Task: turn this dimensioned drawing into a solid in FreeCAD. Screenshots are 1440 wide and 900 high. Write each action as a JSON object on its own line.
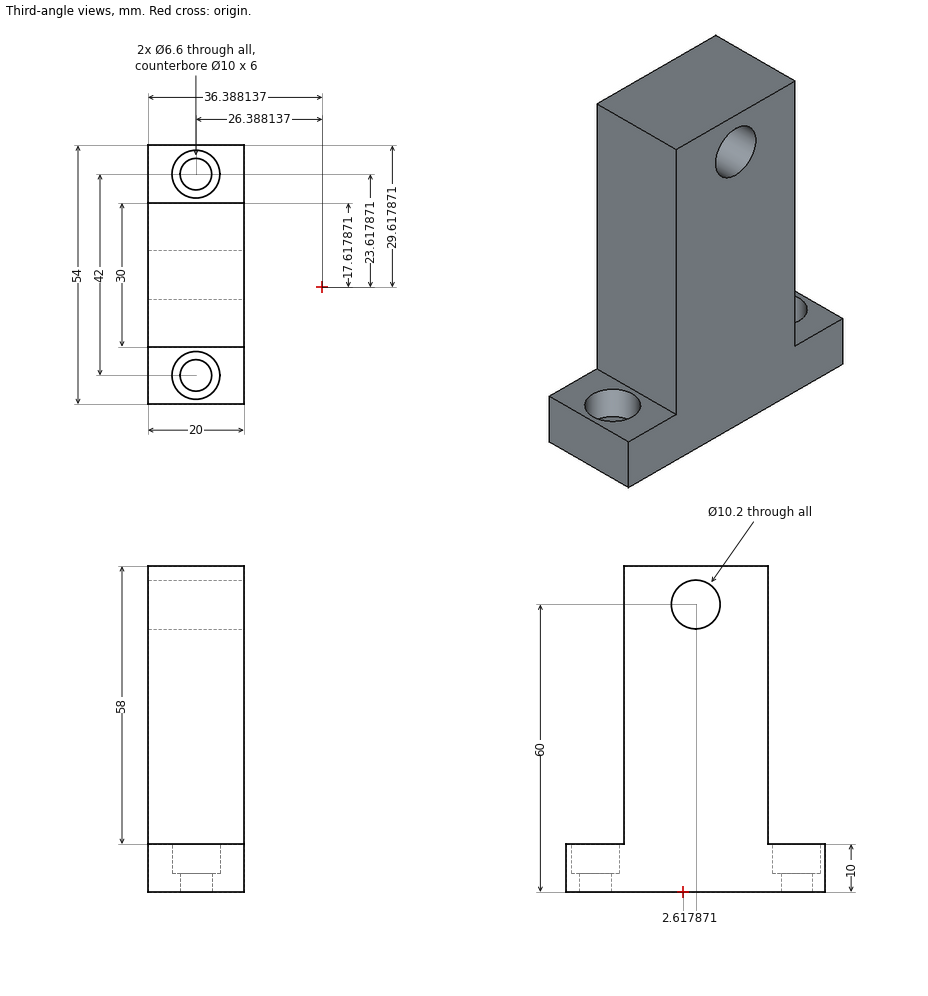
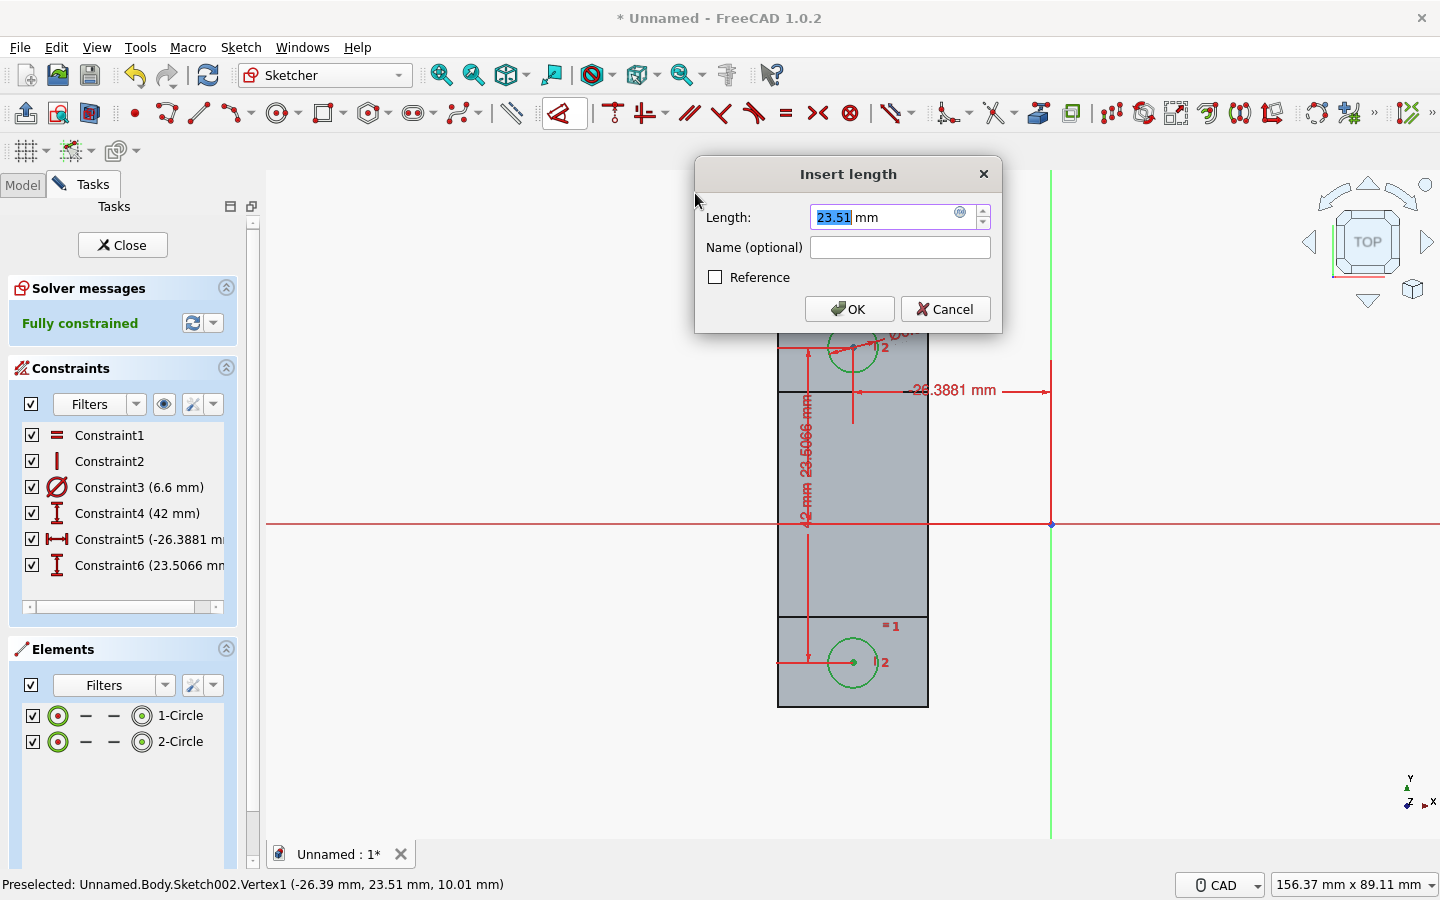
{"action": "type", "text": "23.617871"}
{"action": "key", "text": "Return"}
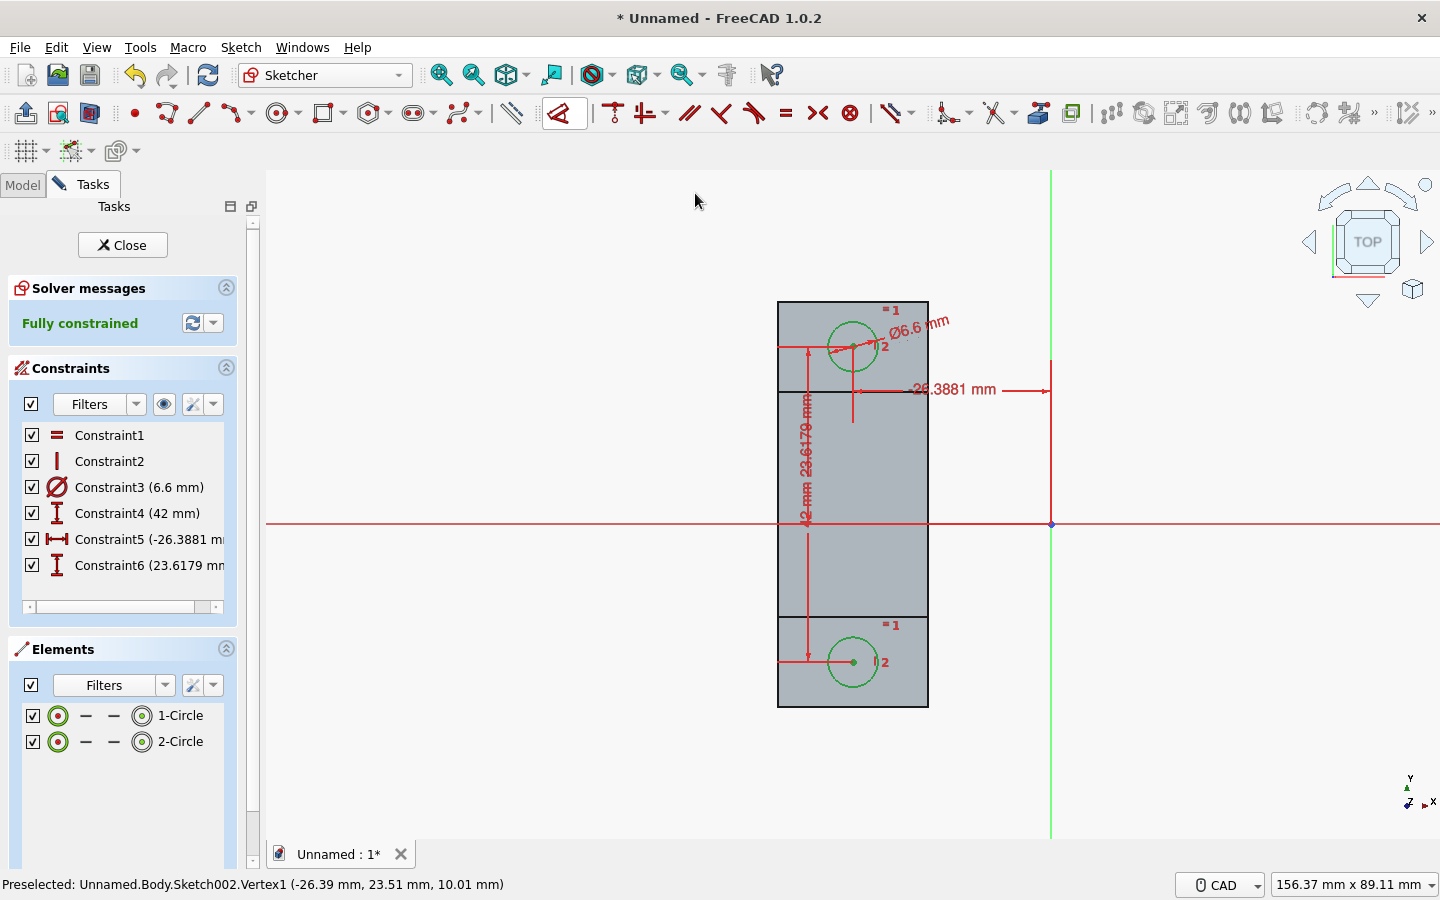
{"action": "left_click", "coordinate": [123, 245]}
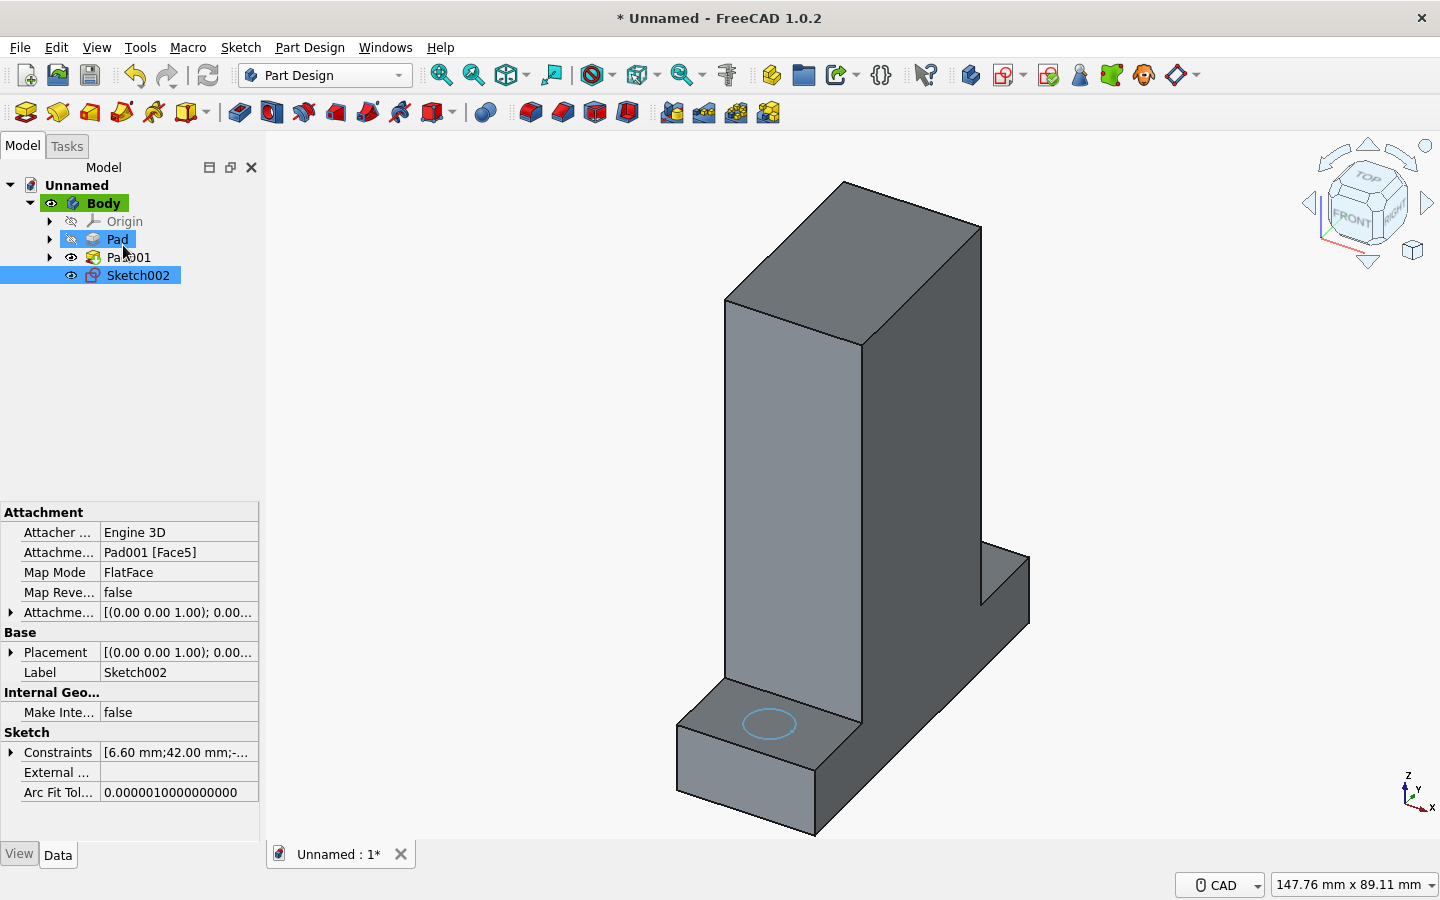
{"action": "left_click", "coordinate": [272, 112]}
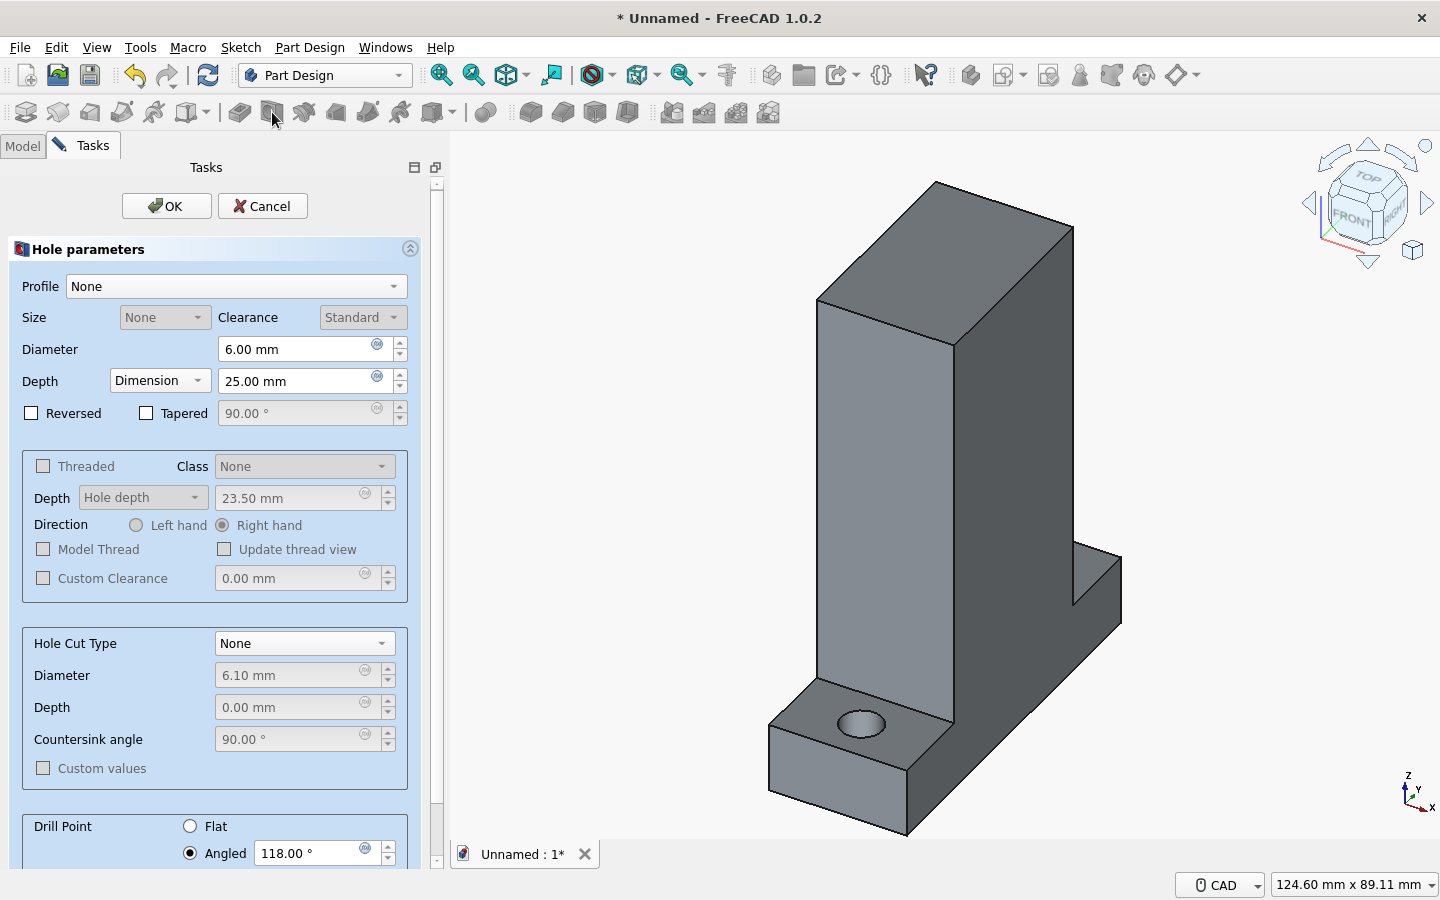
{"action": "triple_click", "coordinate": [305, 349]}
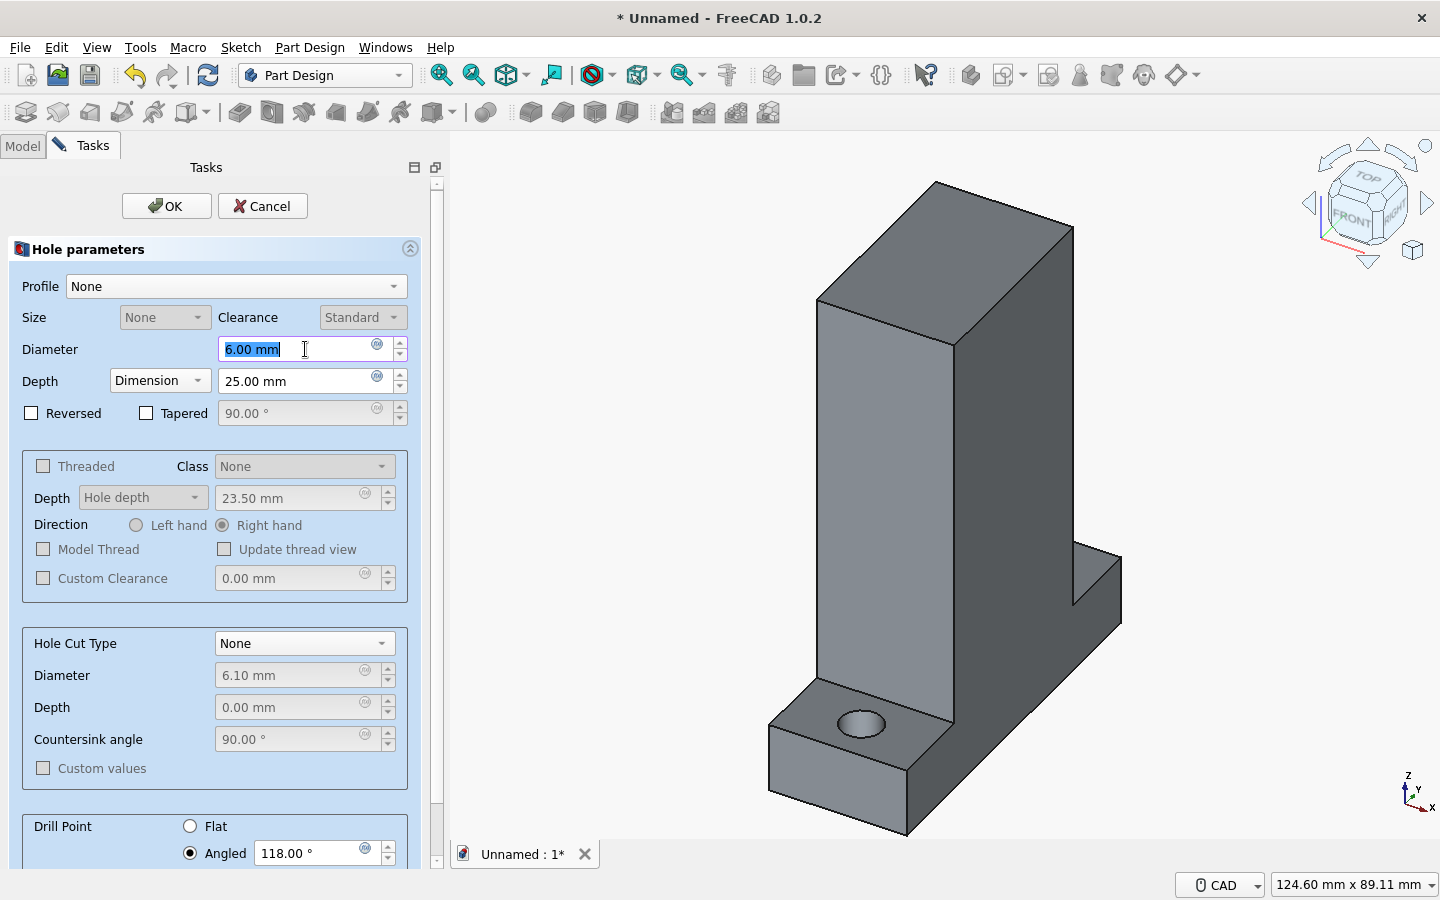
{"action": "type", "text": "6.6"}
{"action": "key", "text": "Tab"}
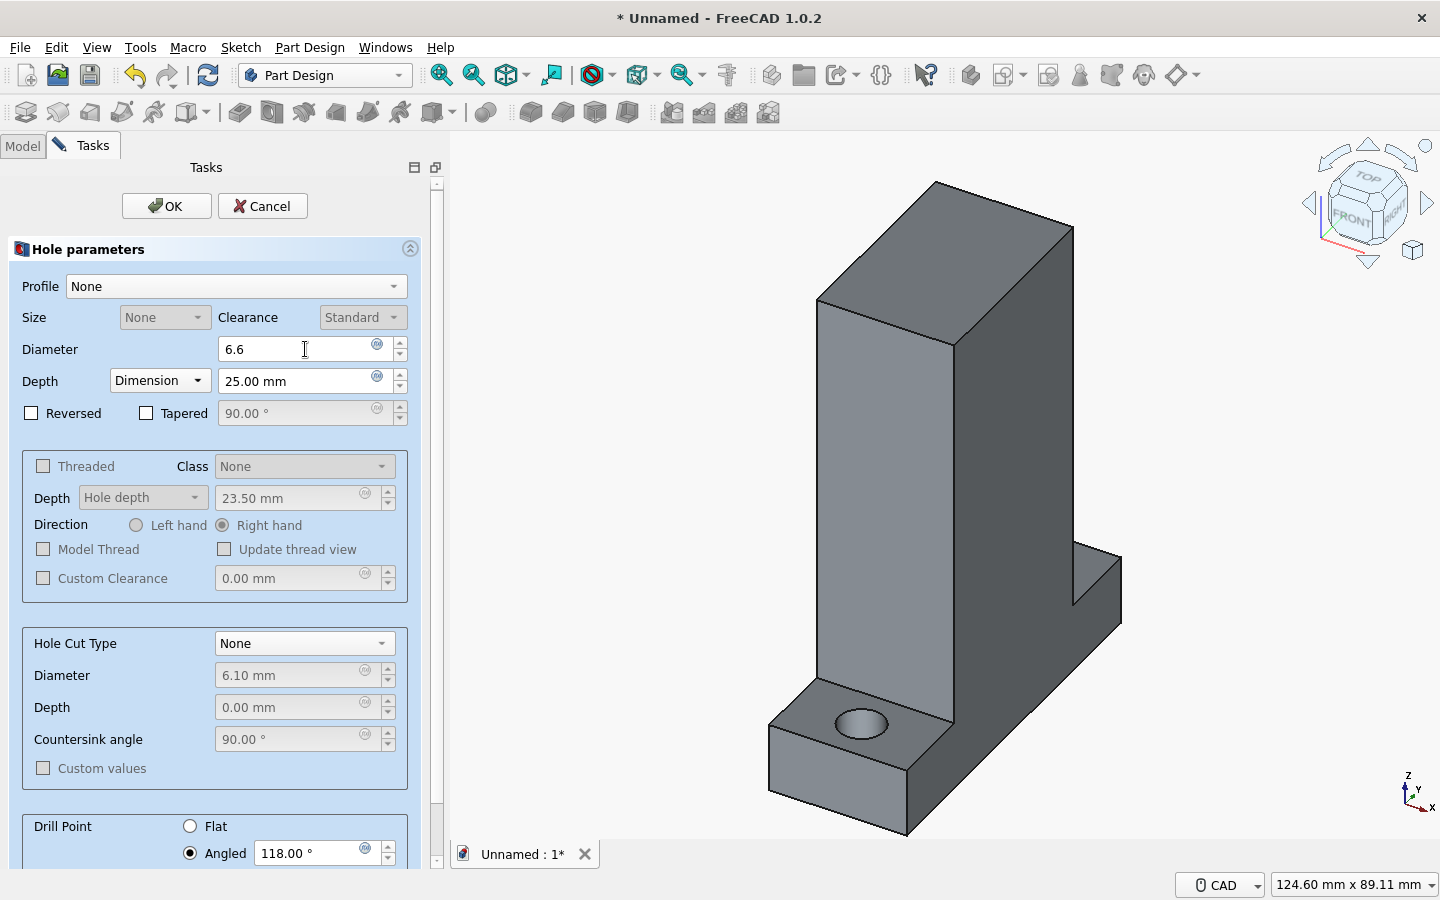
{"action": "left_click", "coordinate": [161, 380]}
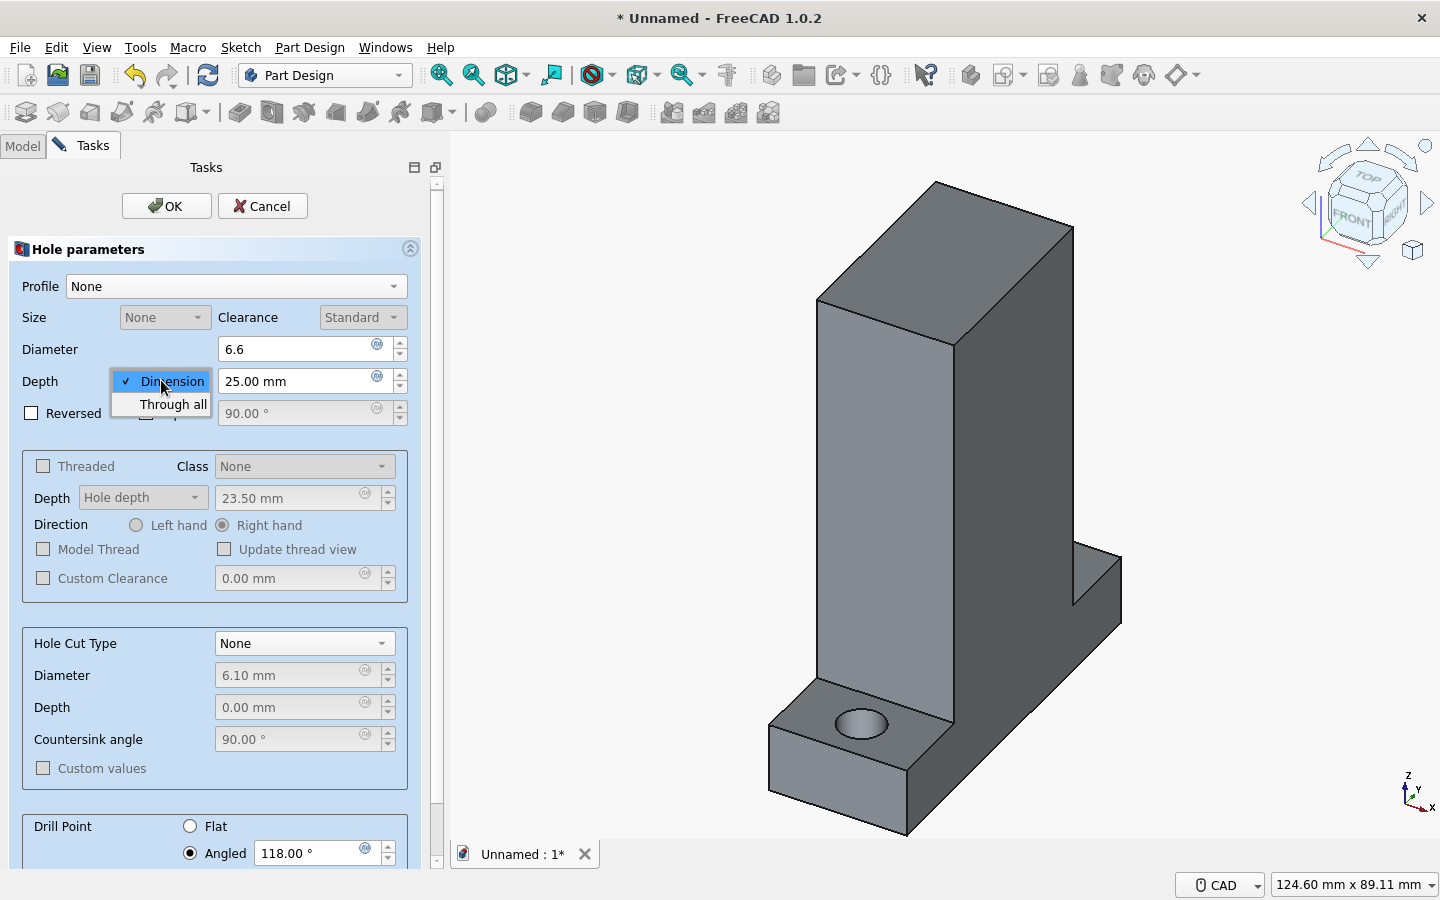
{"action": "left_click", "coordinate": [160, 404]}